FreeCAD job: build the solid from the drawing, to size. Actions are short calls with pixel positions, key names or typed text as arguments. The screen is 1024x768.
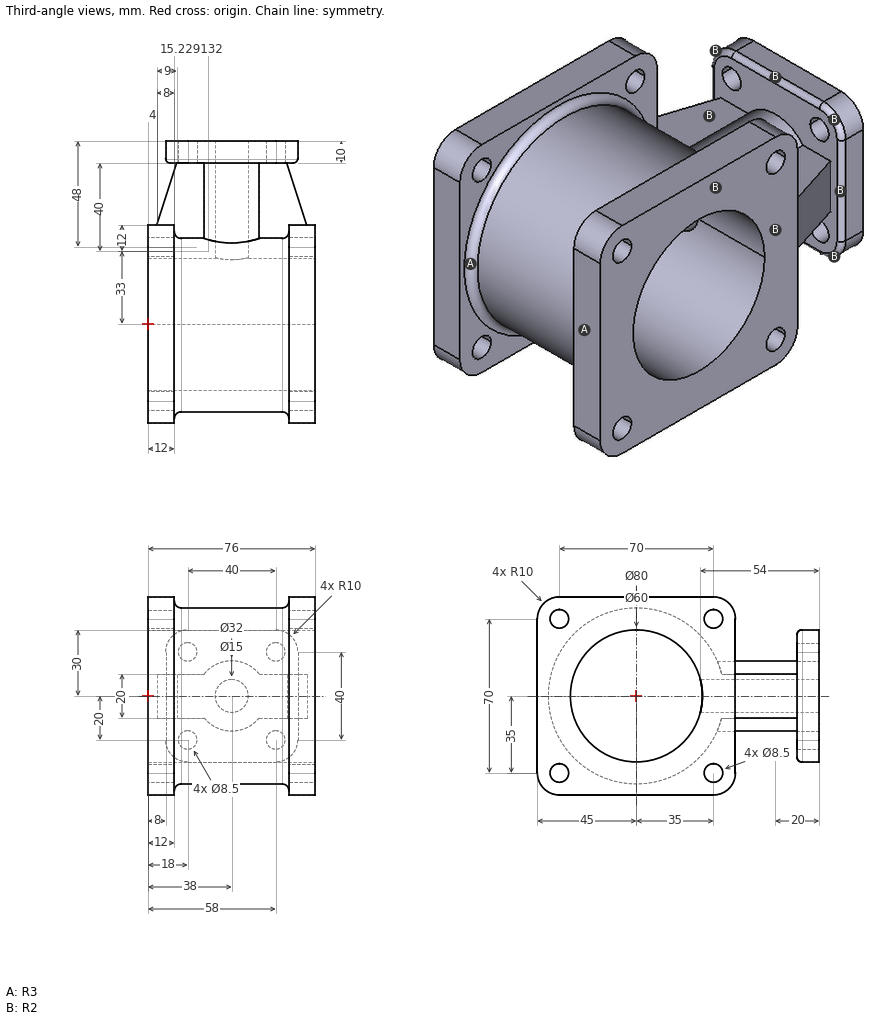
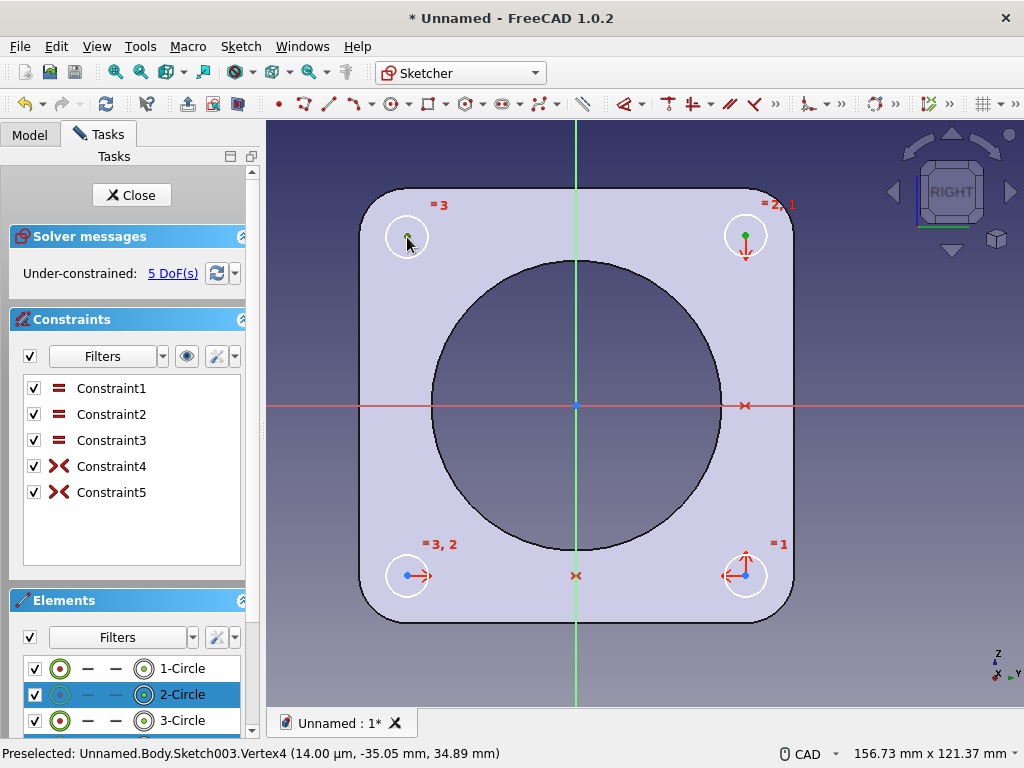
click(577, 641)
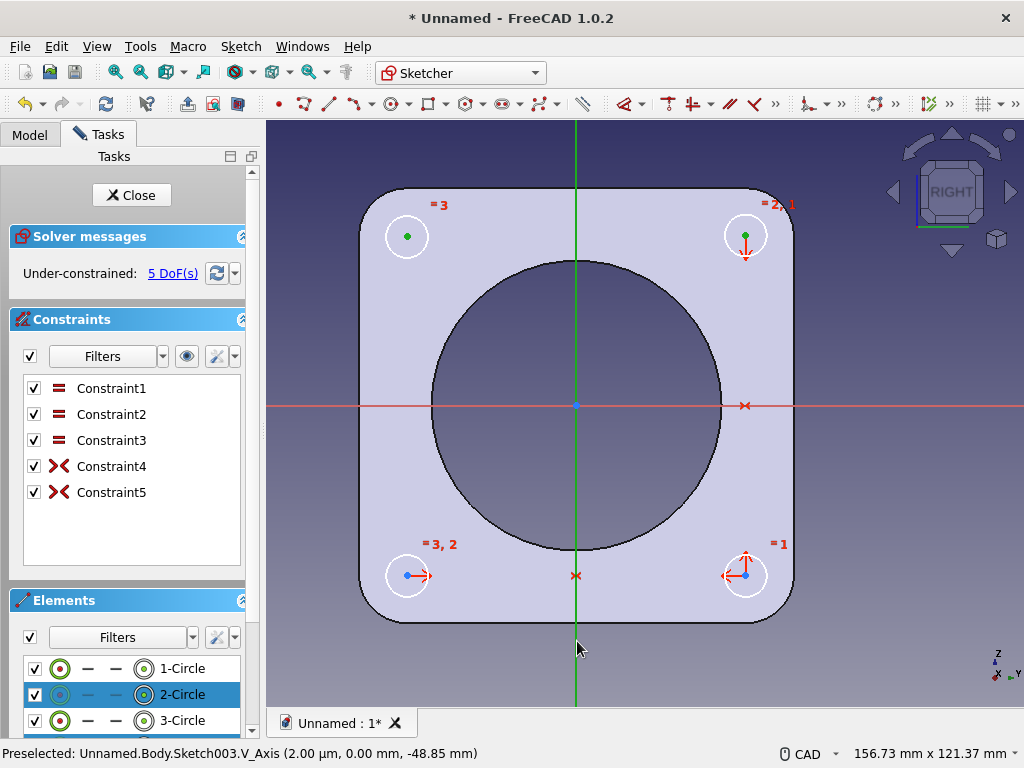
key(s)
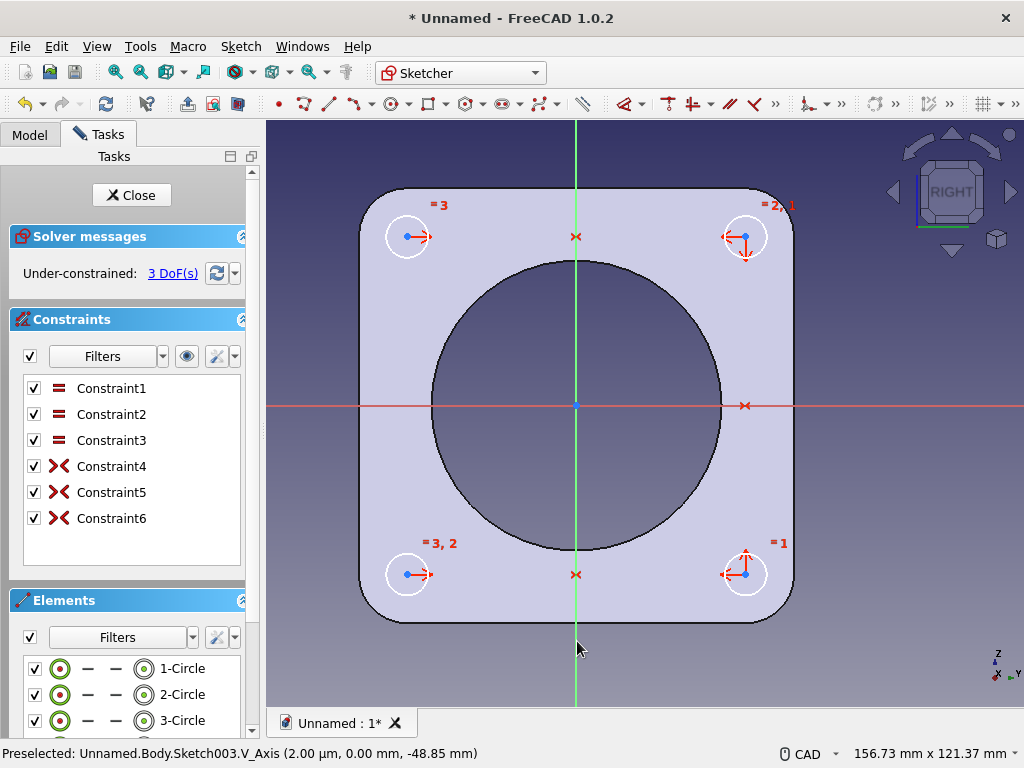
click(624, 104)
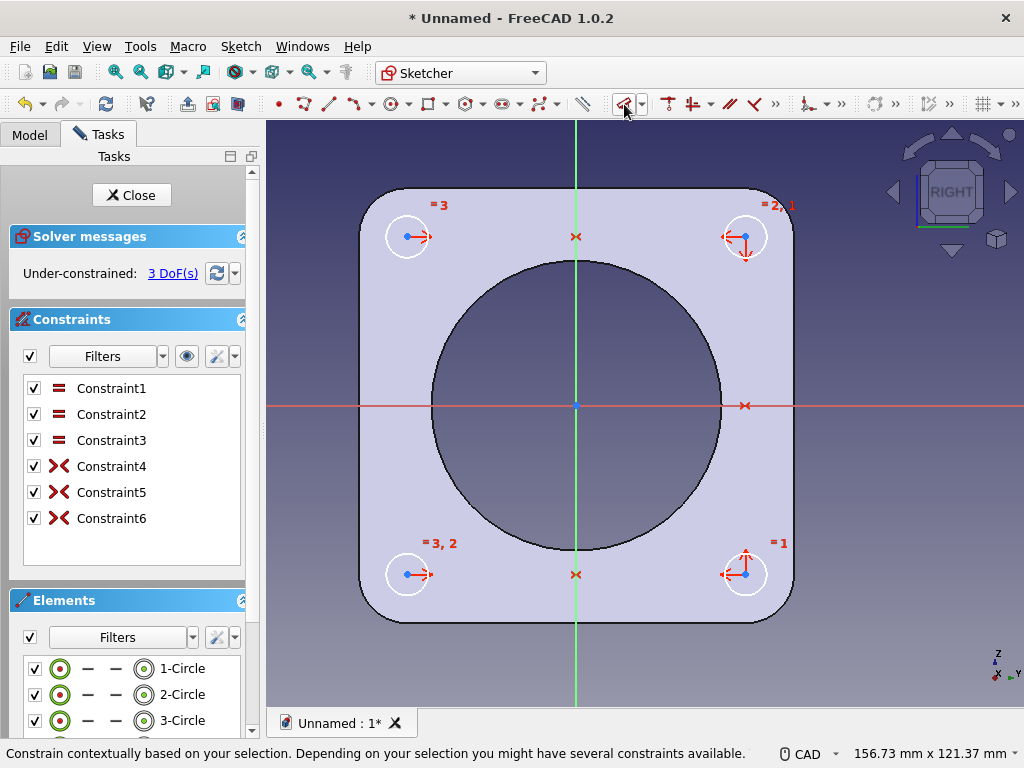
click(761, 560)
click(784, 538)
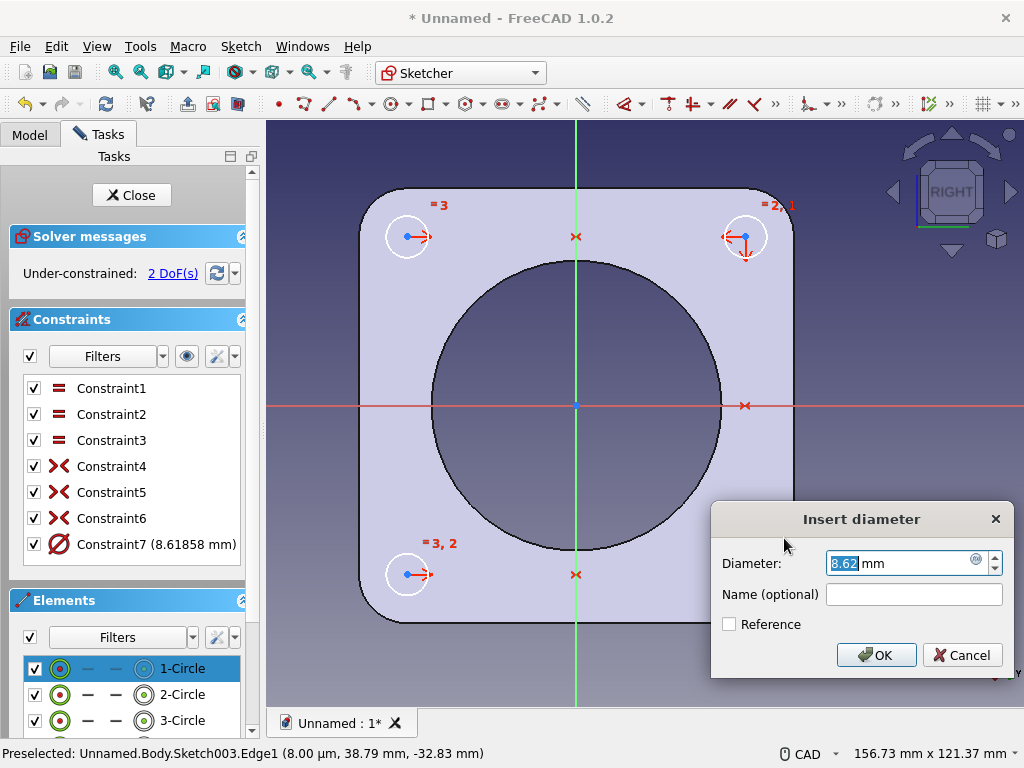
text(8.5)
key(Return)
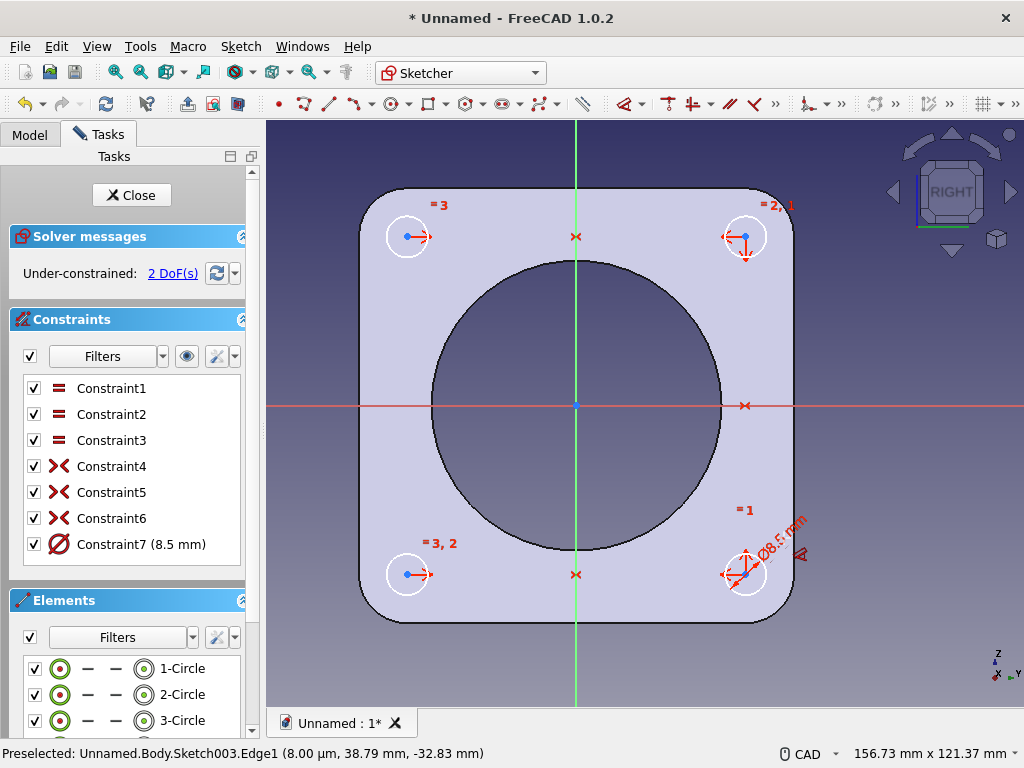
click(746, 575)
click(661, 609)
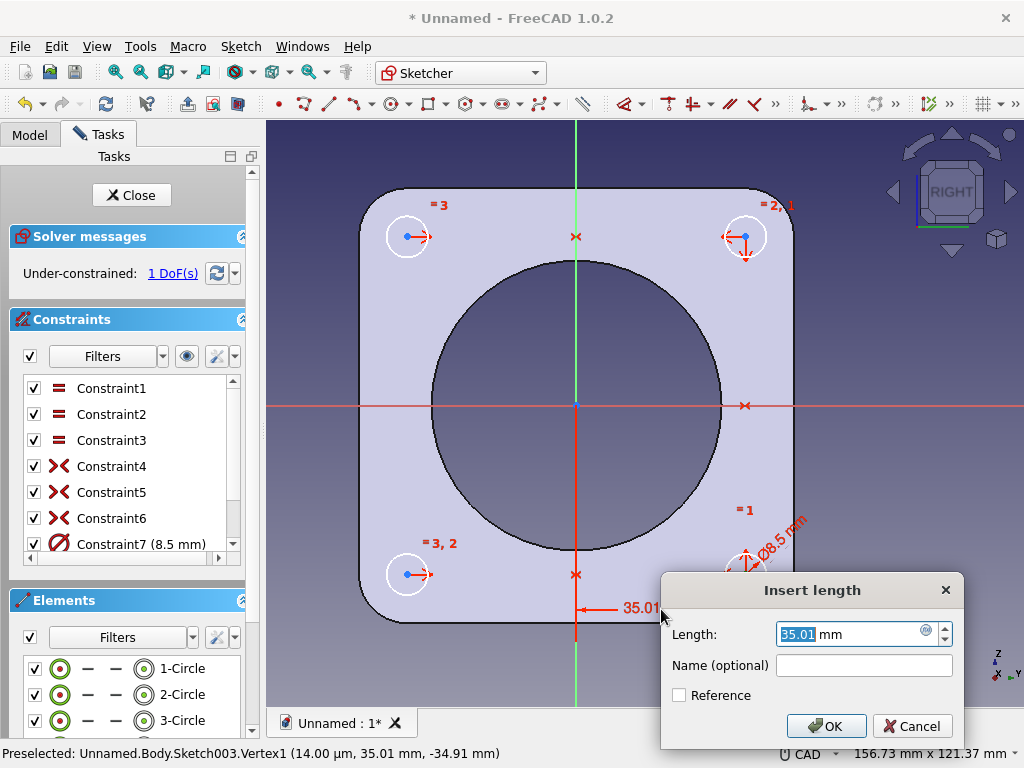
text(35)
key(Return)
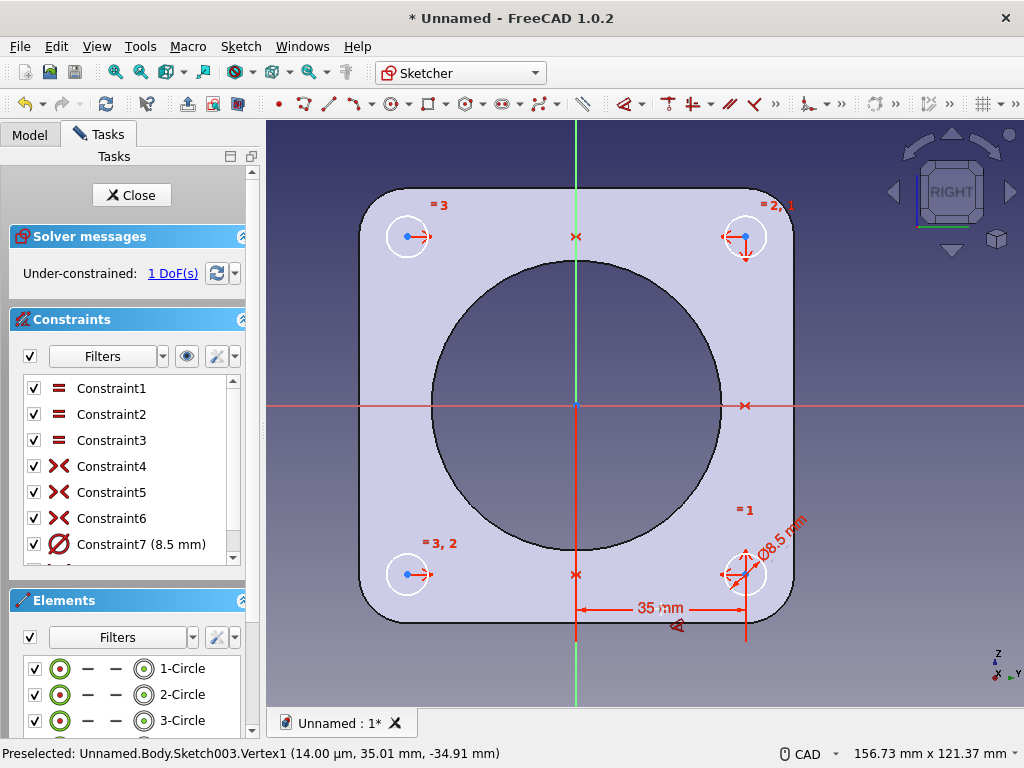
click(746, 575)
click(780, 490)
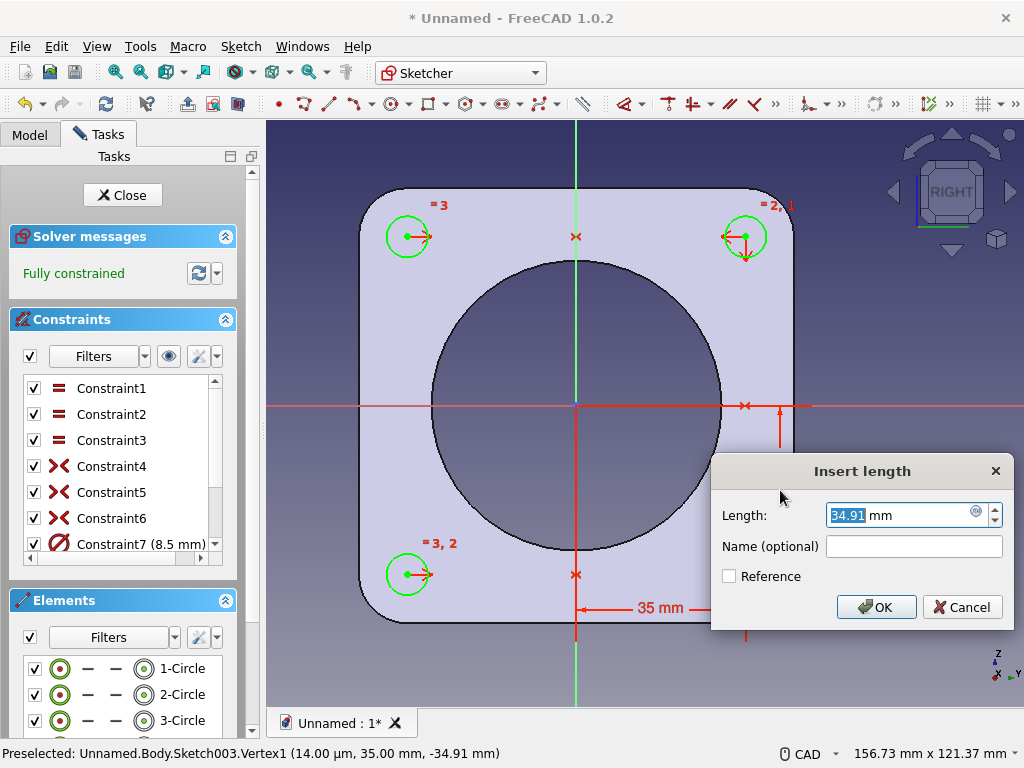
text(35)
key(Return)
key(Escape)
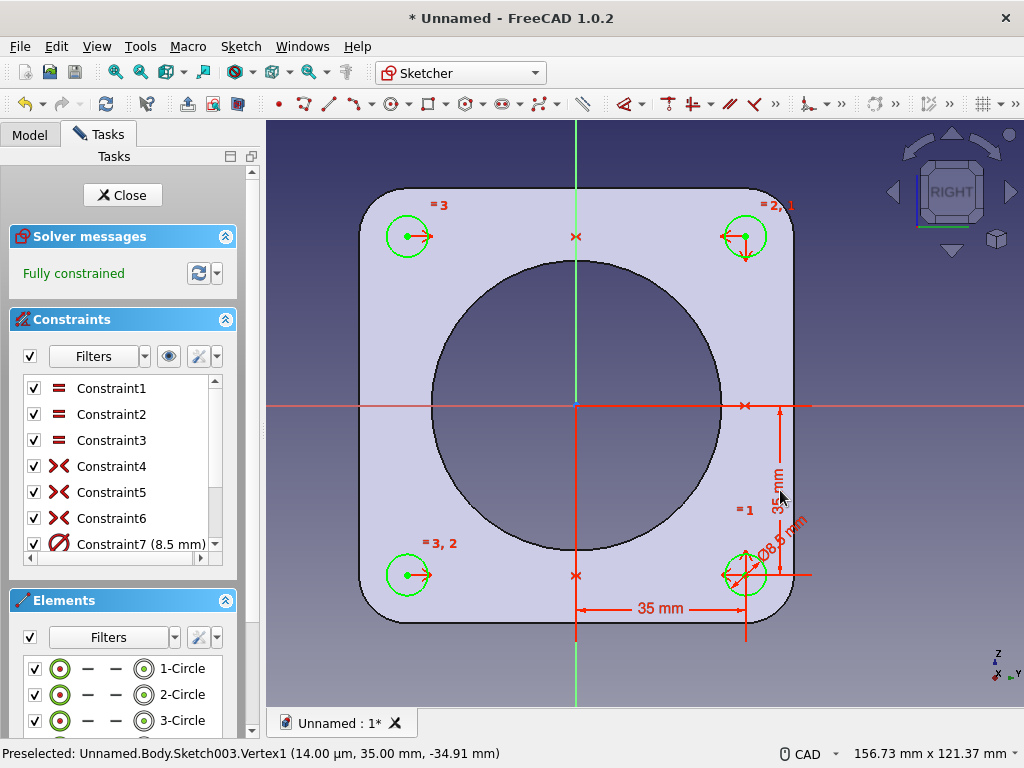
click(123, 195)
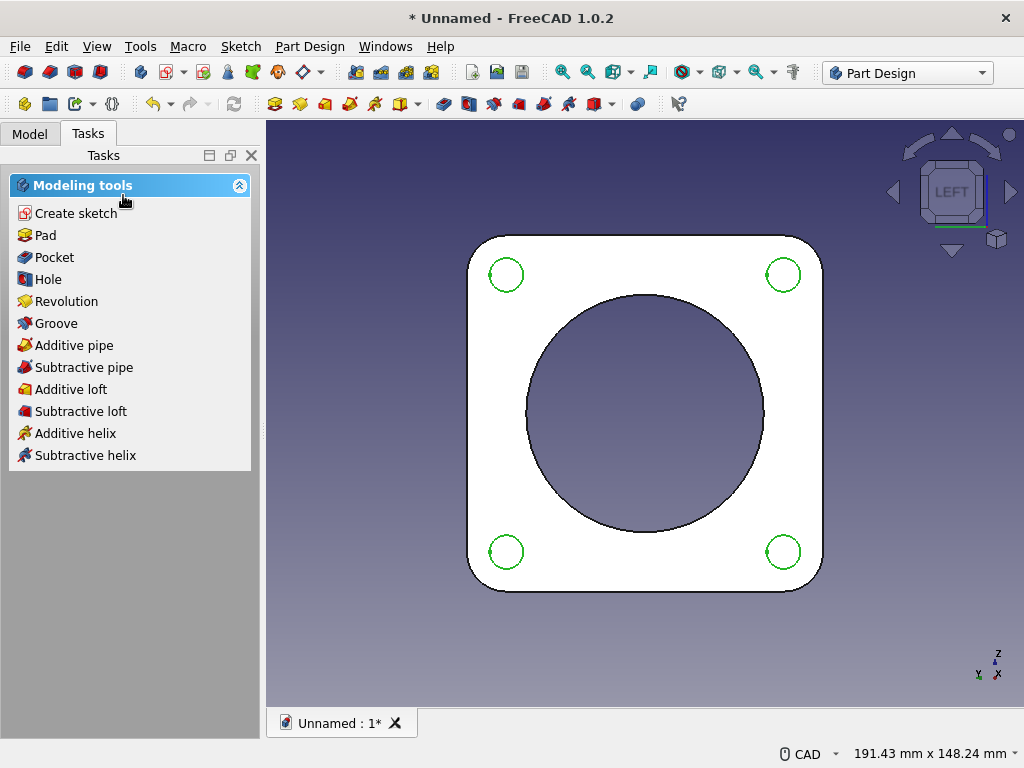
click(444, 104)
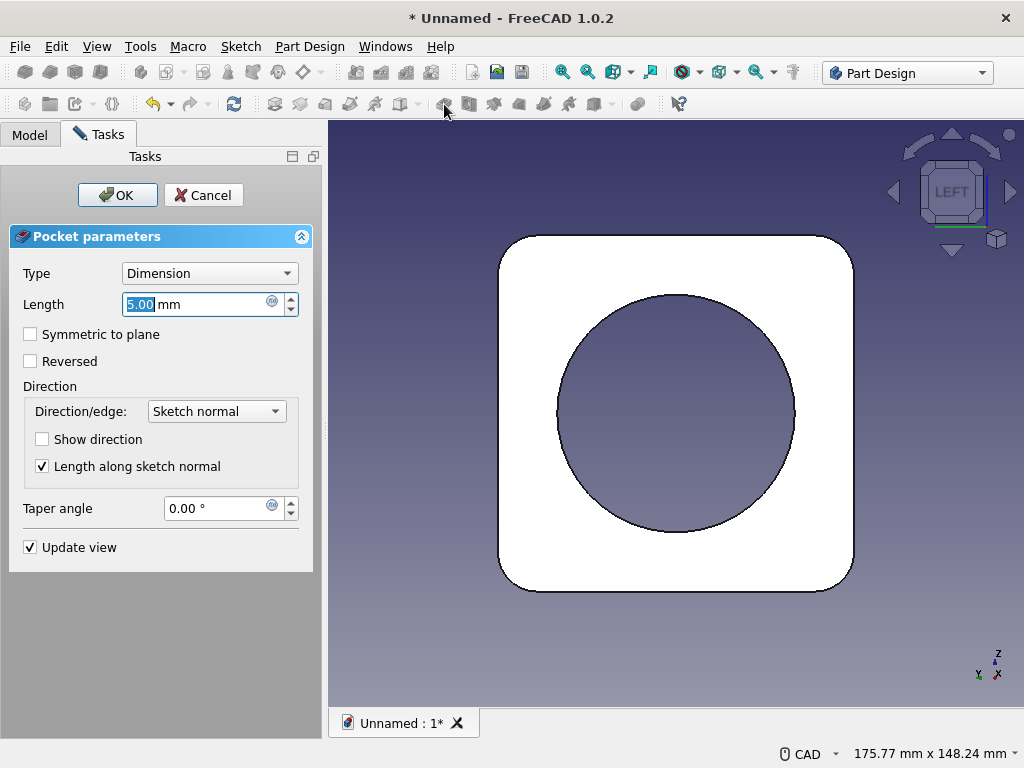
text(12)
key(Tab)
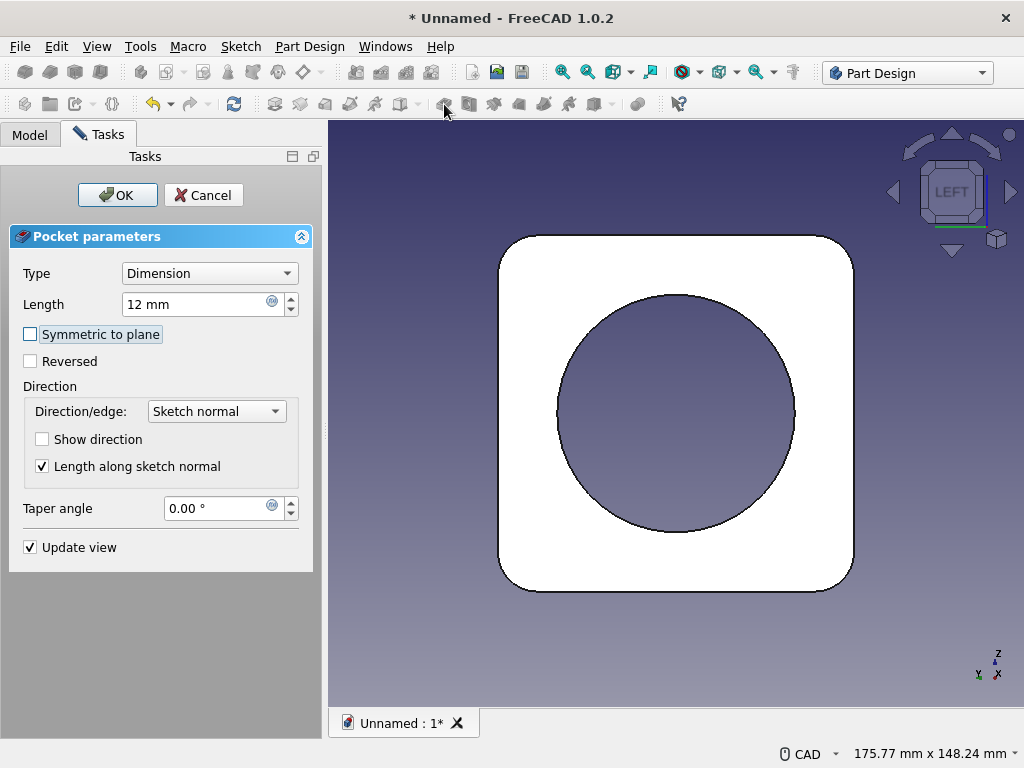
click(31, 361)